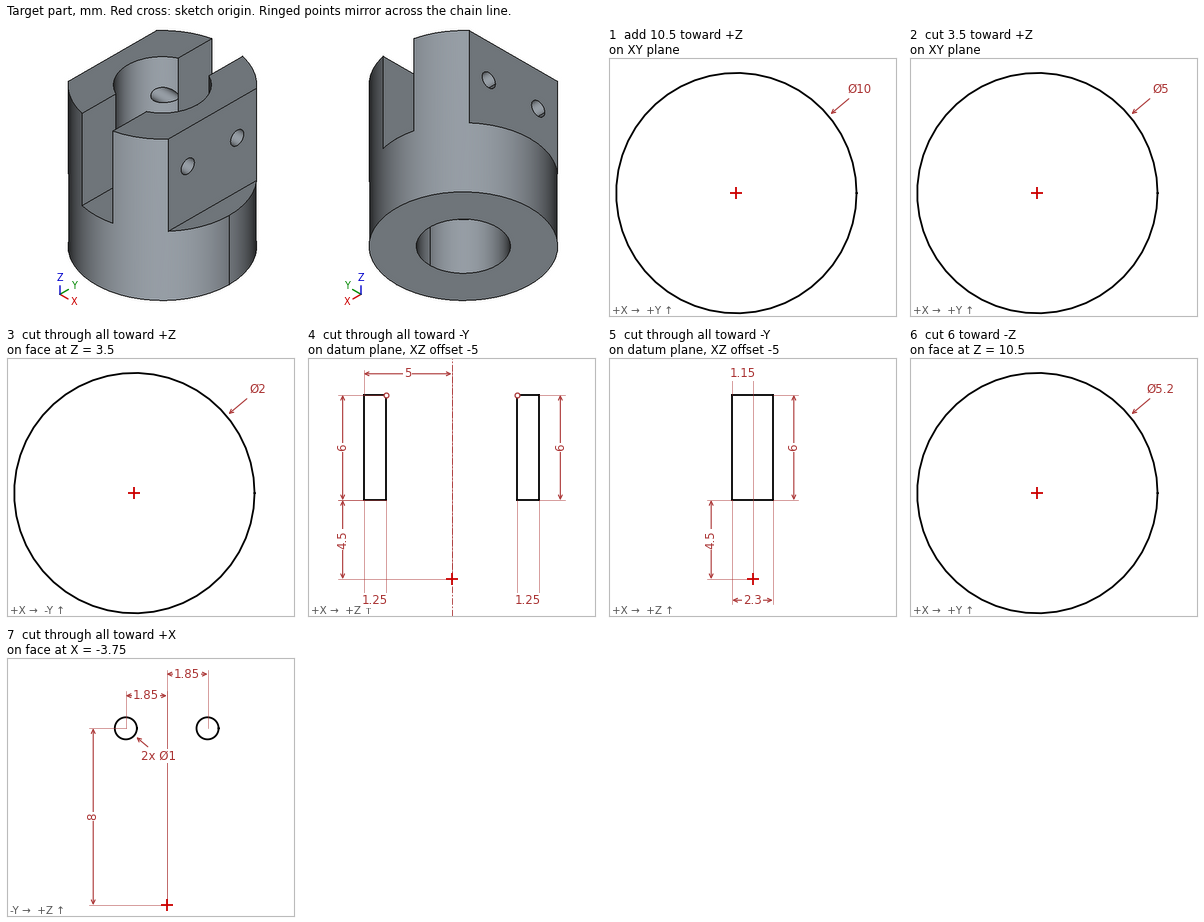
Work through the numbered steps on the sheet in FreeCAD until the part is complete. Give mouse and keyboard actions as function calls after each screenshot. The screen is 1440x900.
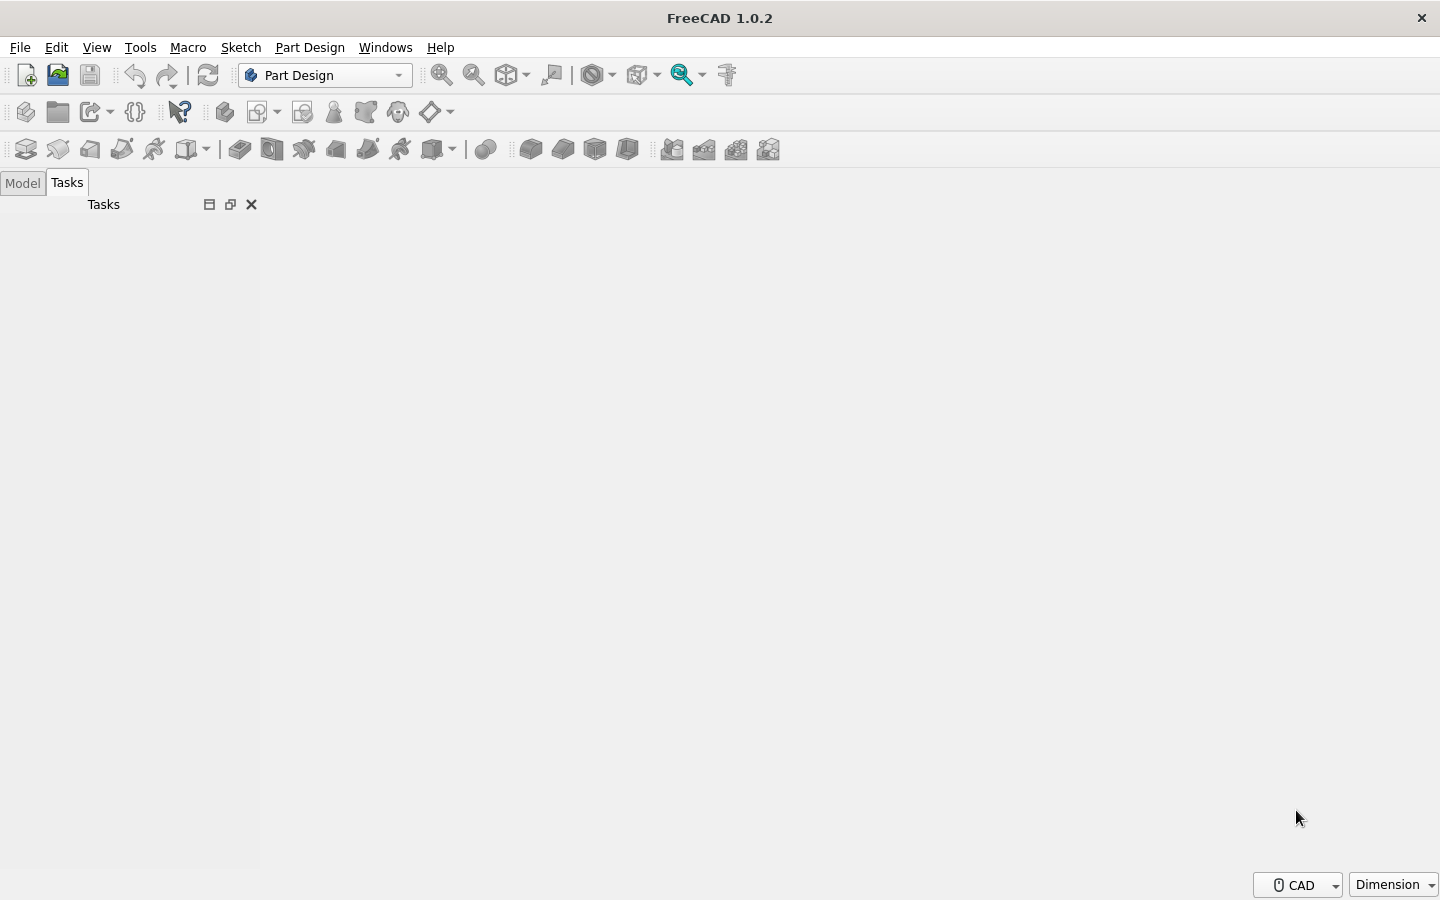
key(ctrl+n)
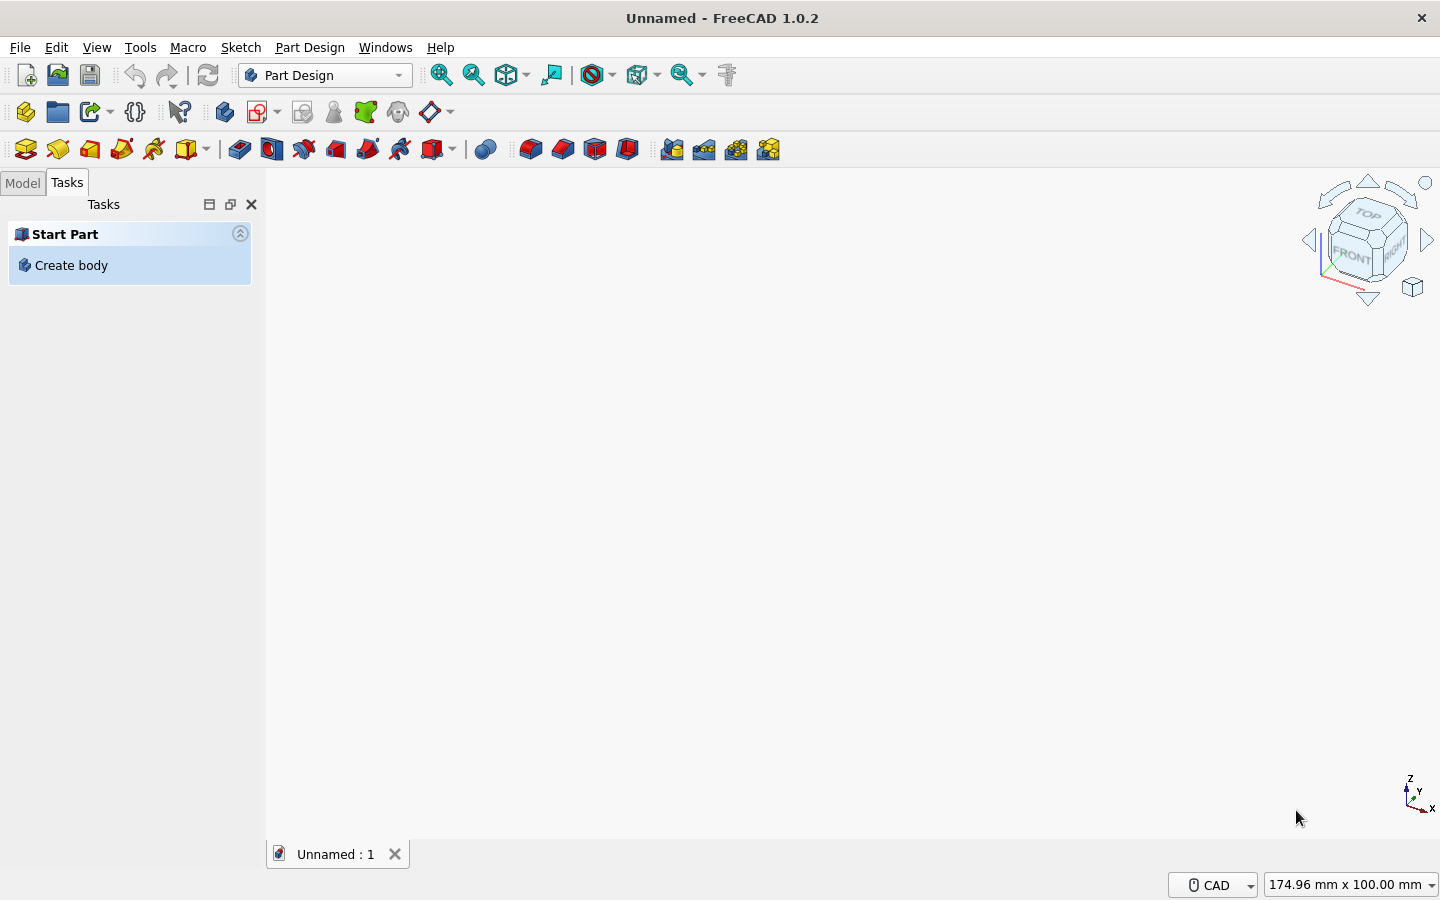
click(258, 112)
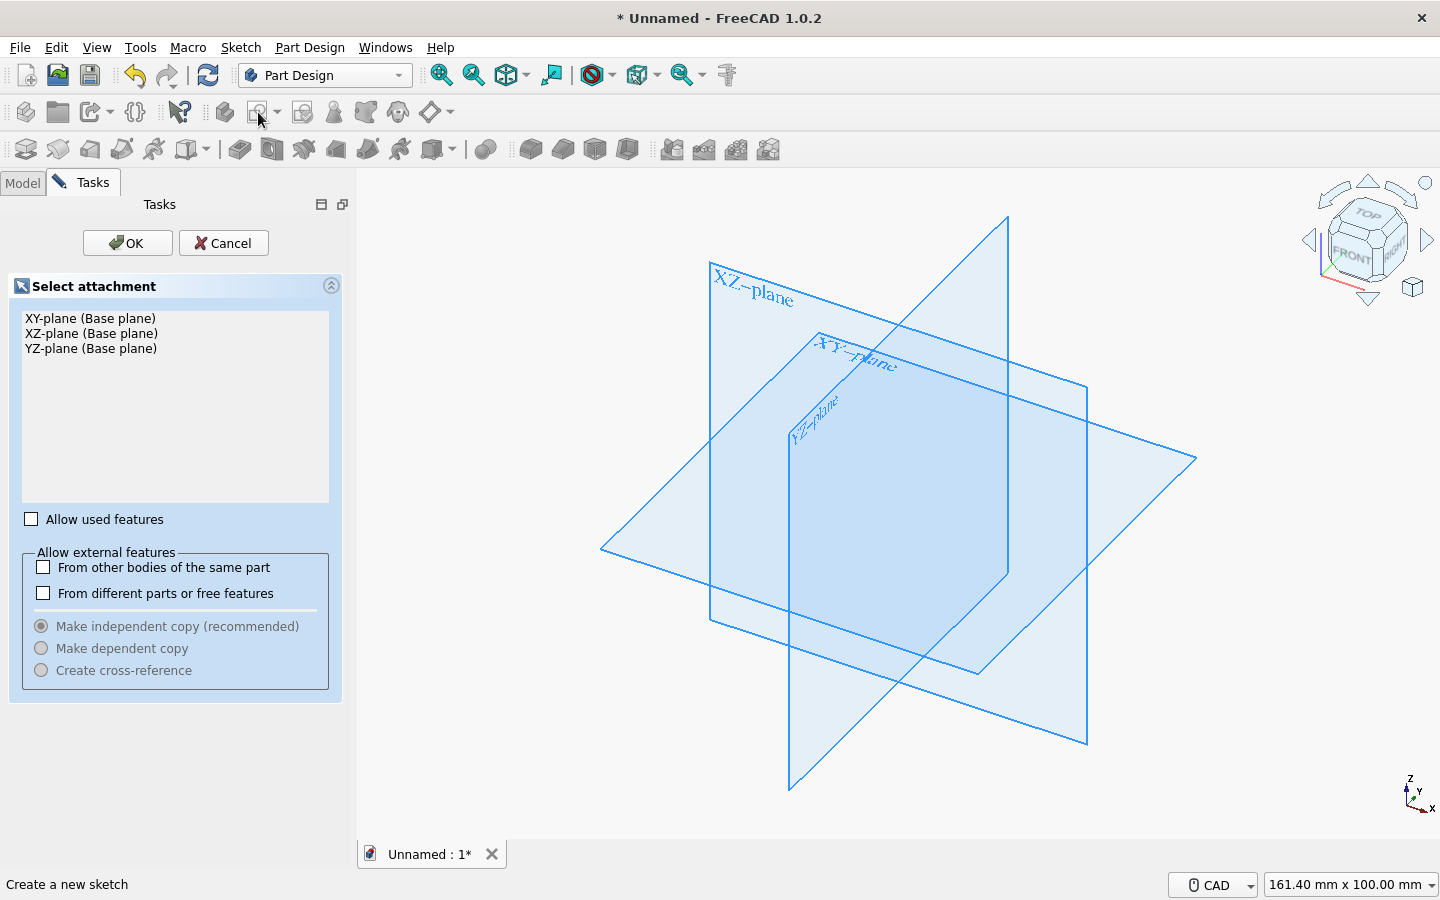
click(82, 318)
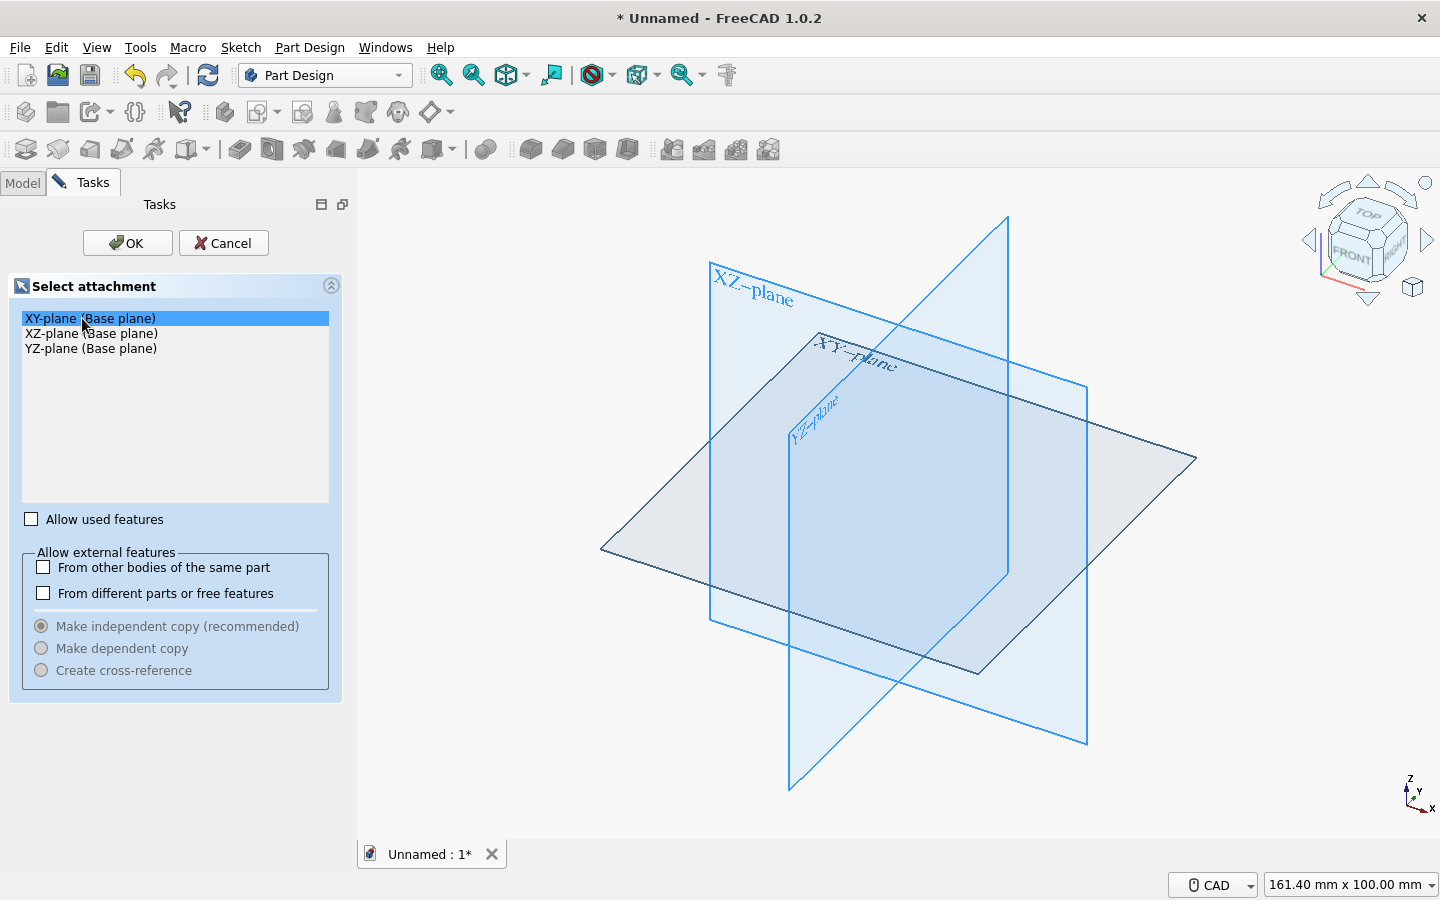
click(128, 243)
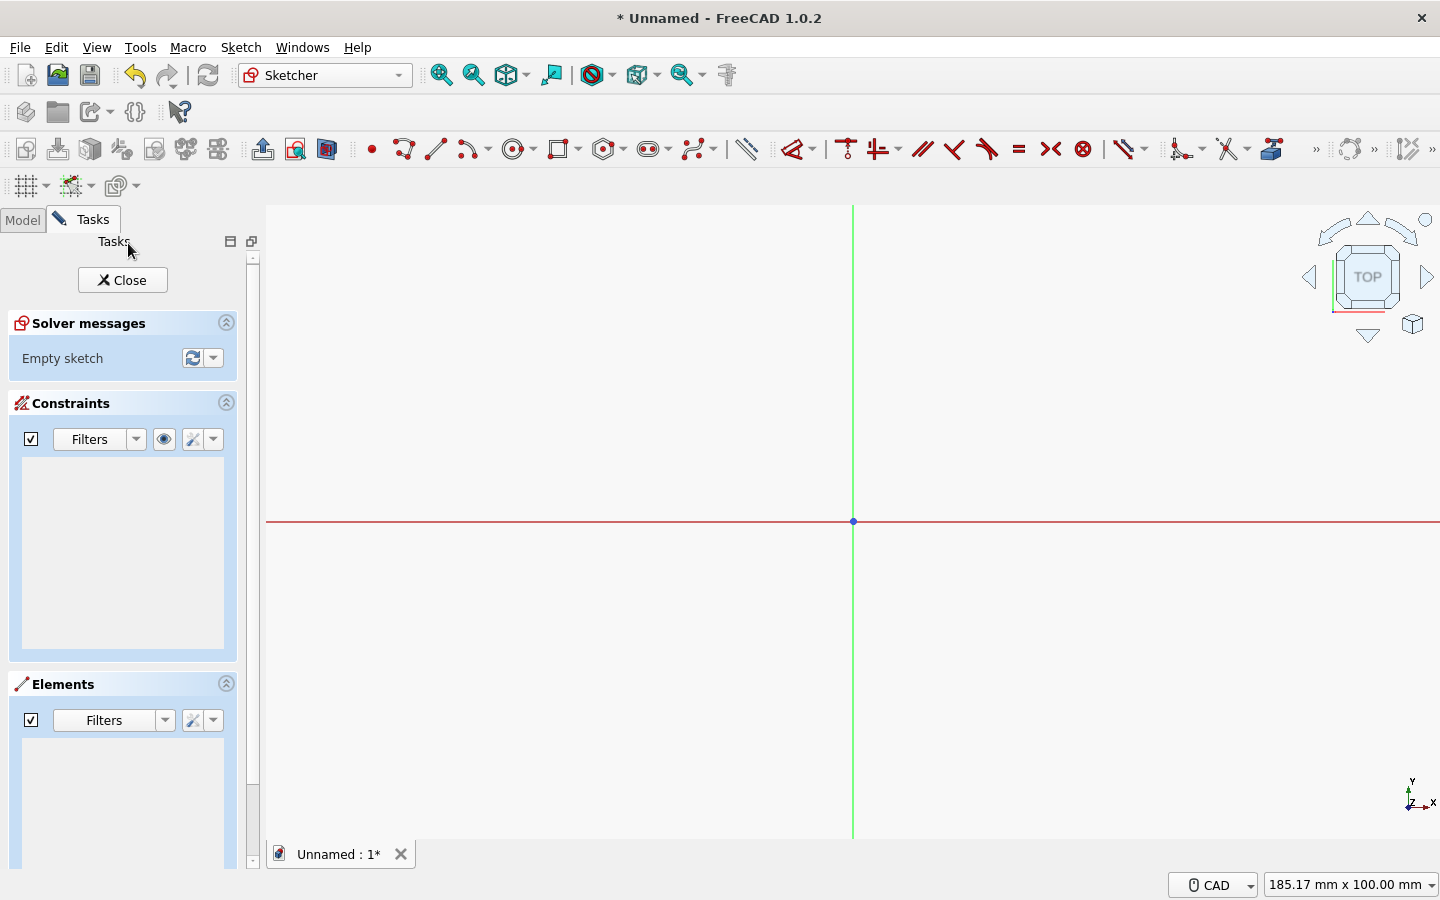
scroll(867, 522, up, 9)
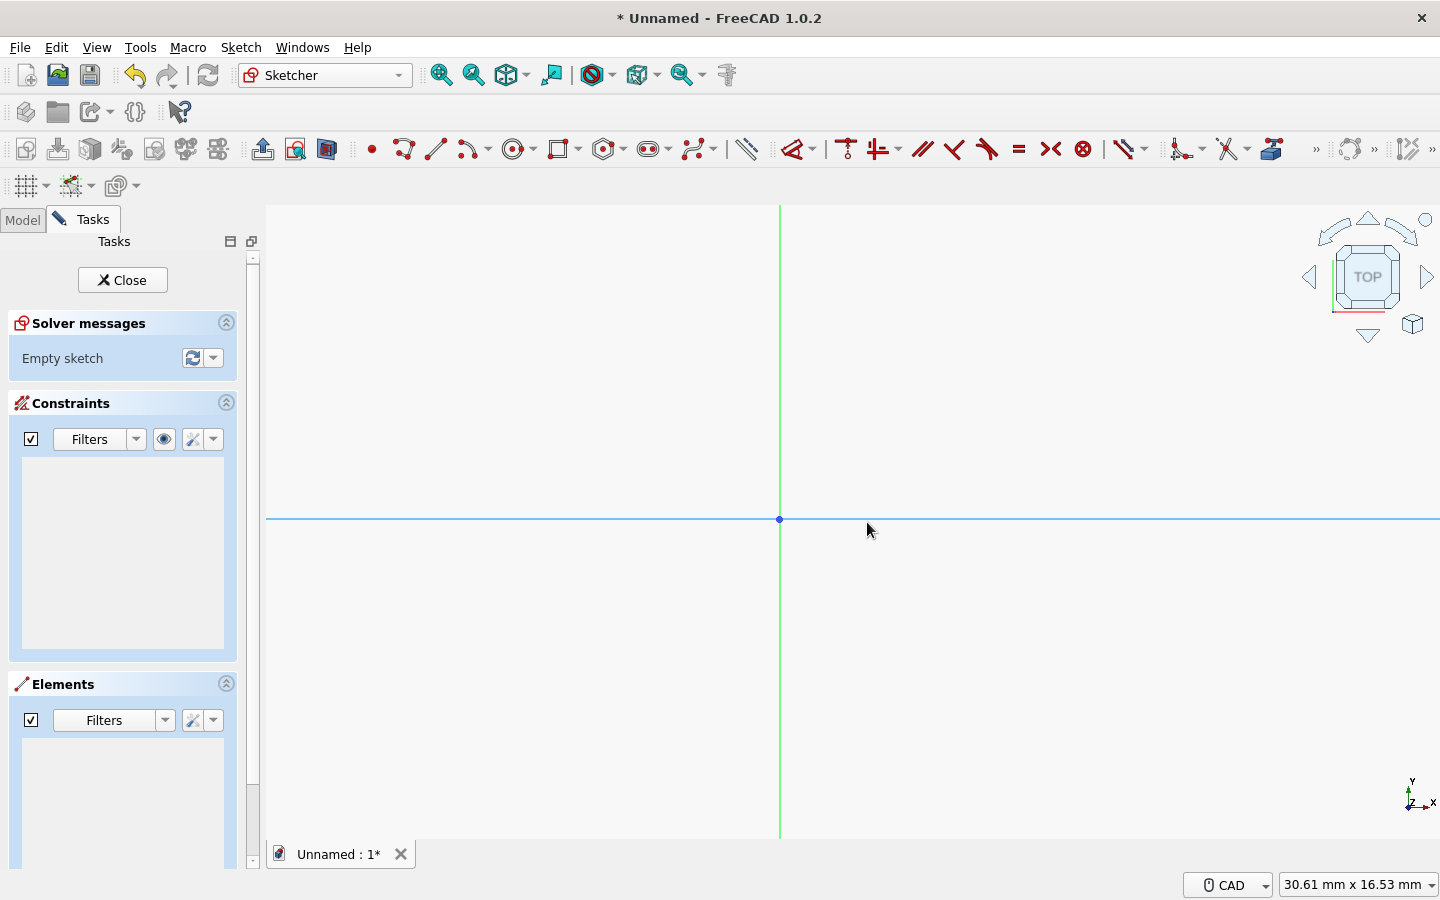
key(g)
key(c)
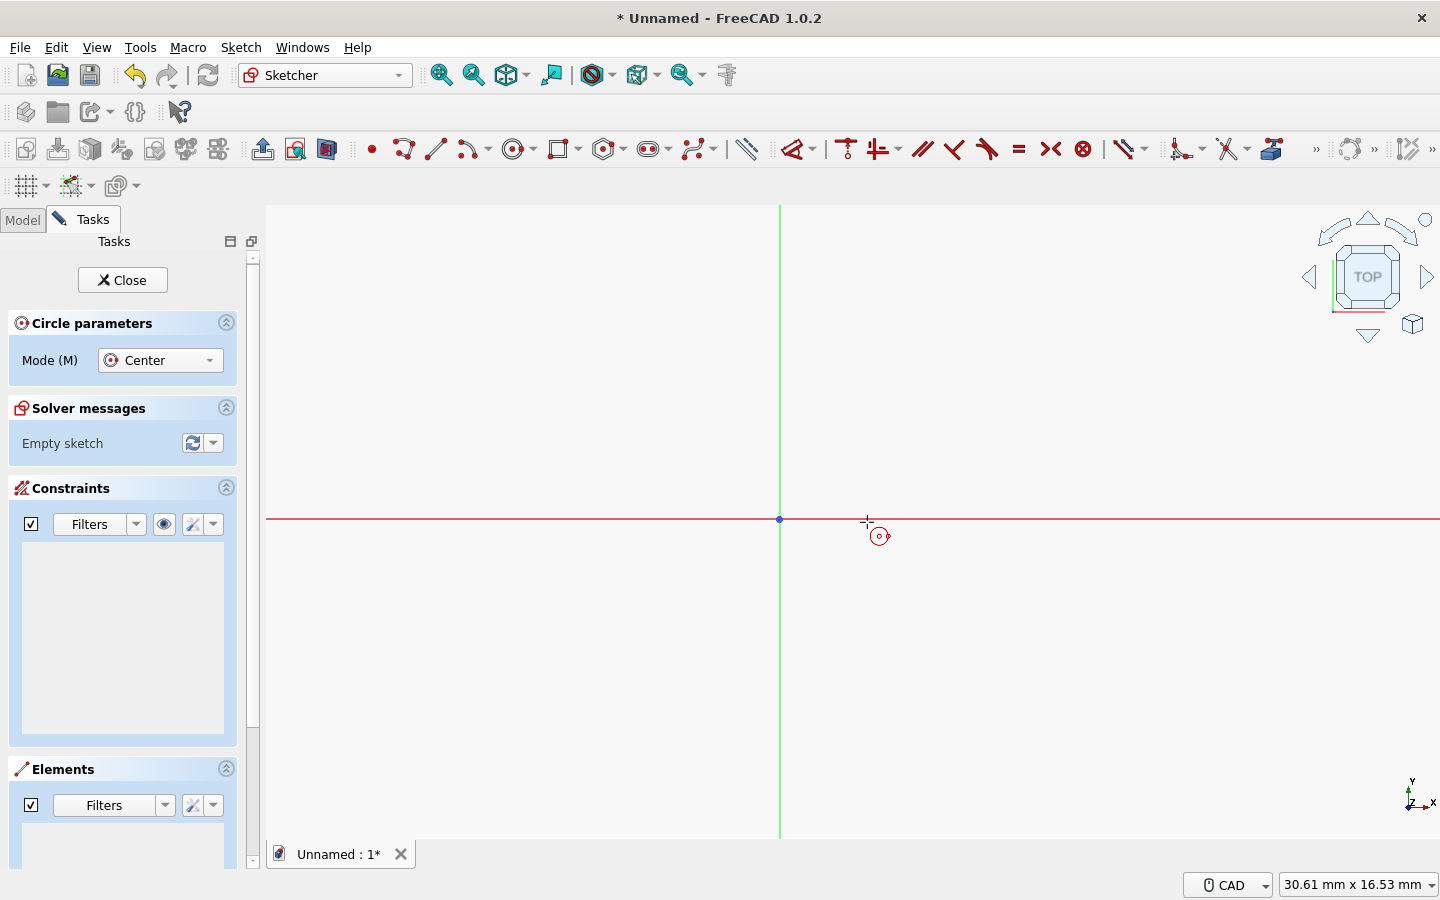
click(780, 519)
move(915, 384)